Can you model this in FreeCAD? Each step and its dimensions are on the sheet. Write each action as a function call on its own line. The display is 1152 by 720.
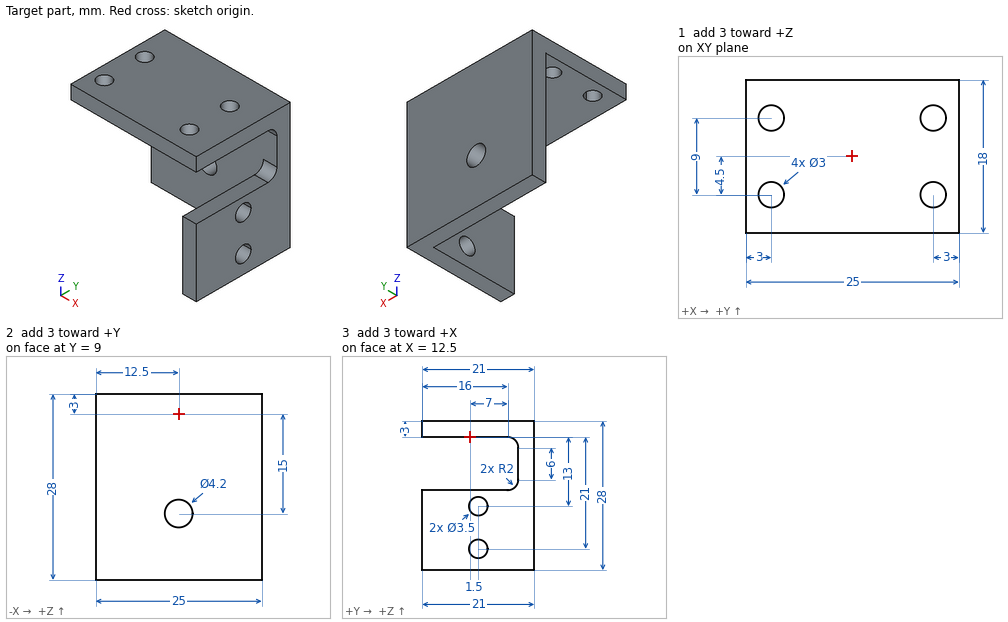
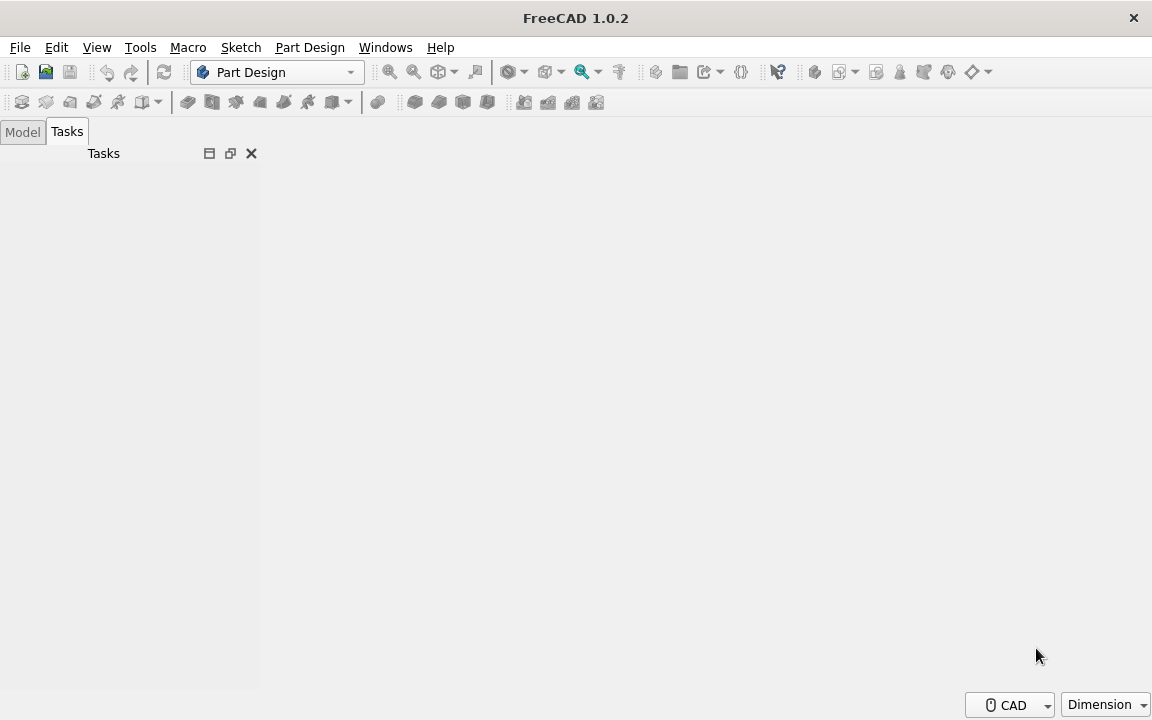
key(ctrl+n)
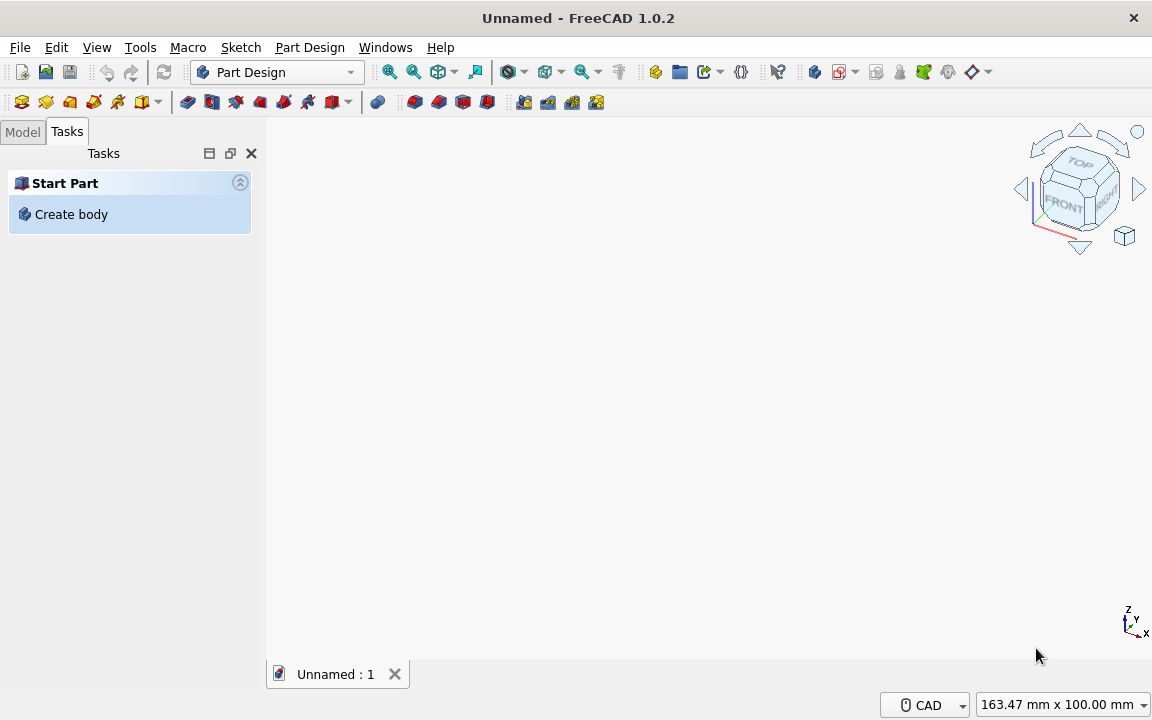
click(840, 72)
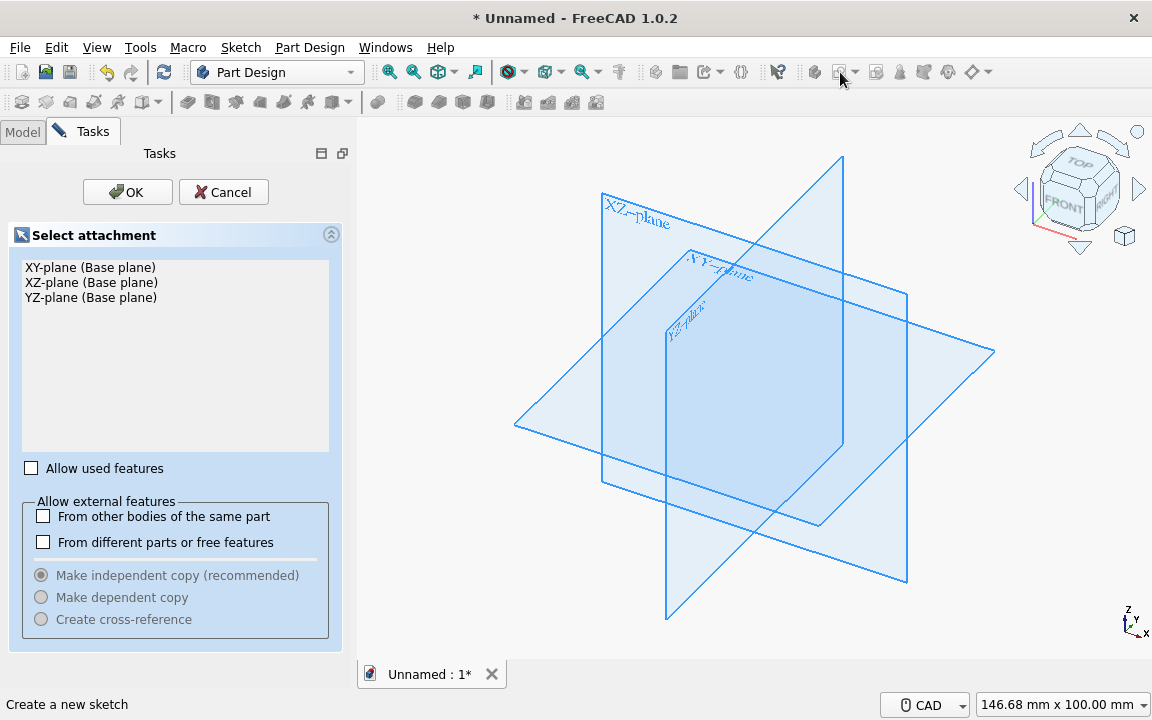
click(82, 268)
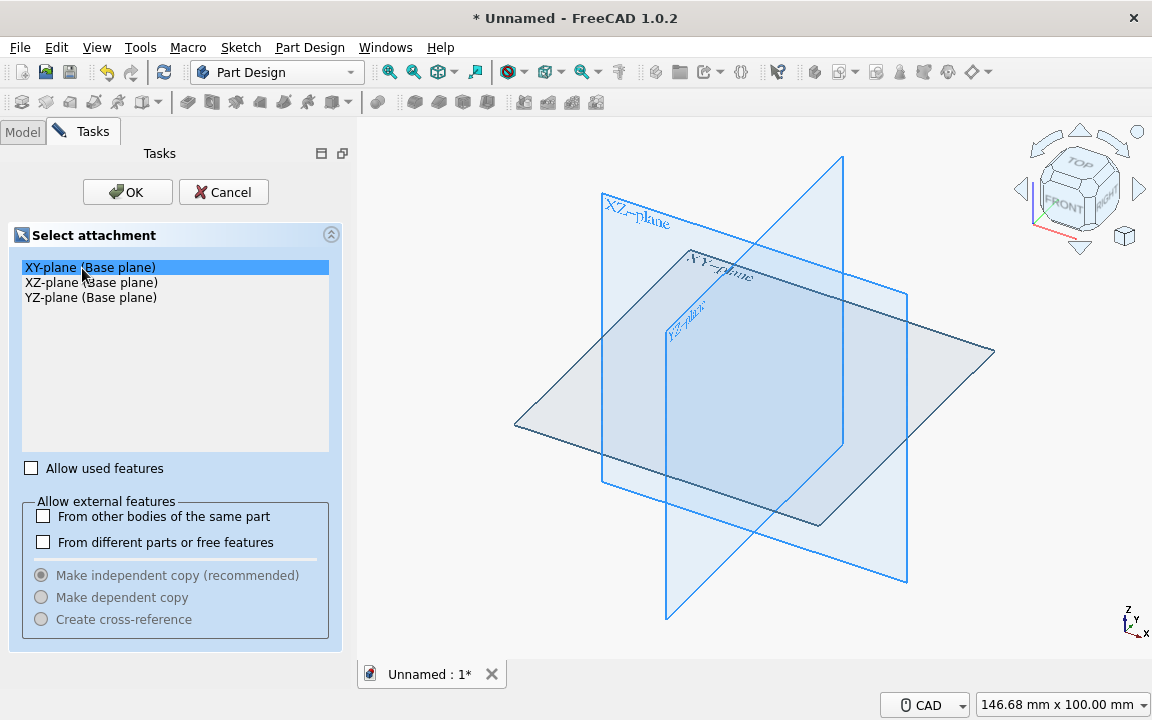
click(128, 192)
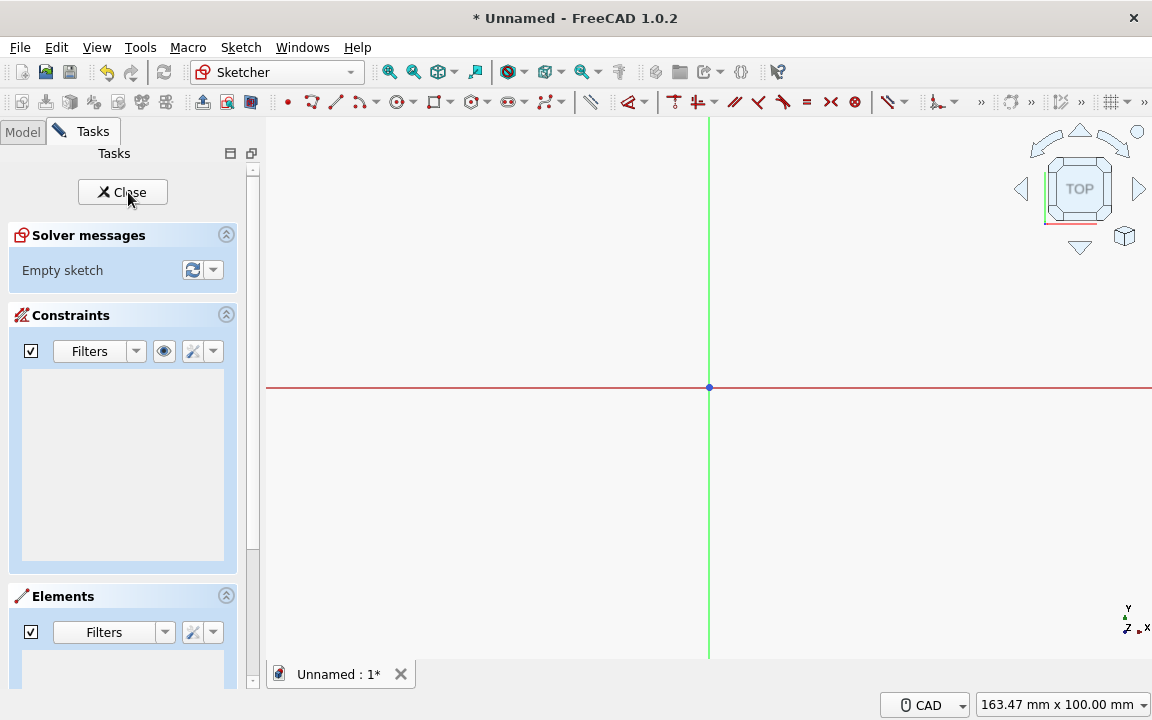
scroll(739, 388, up, 6)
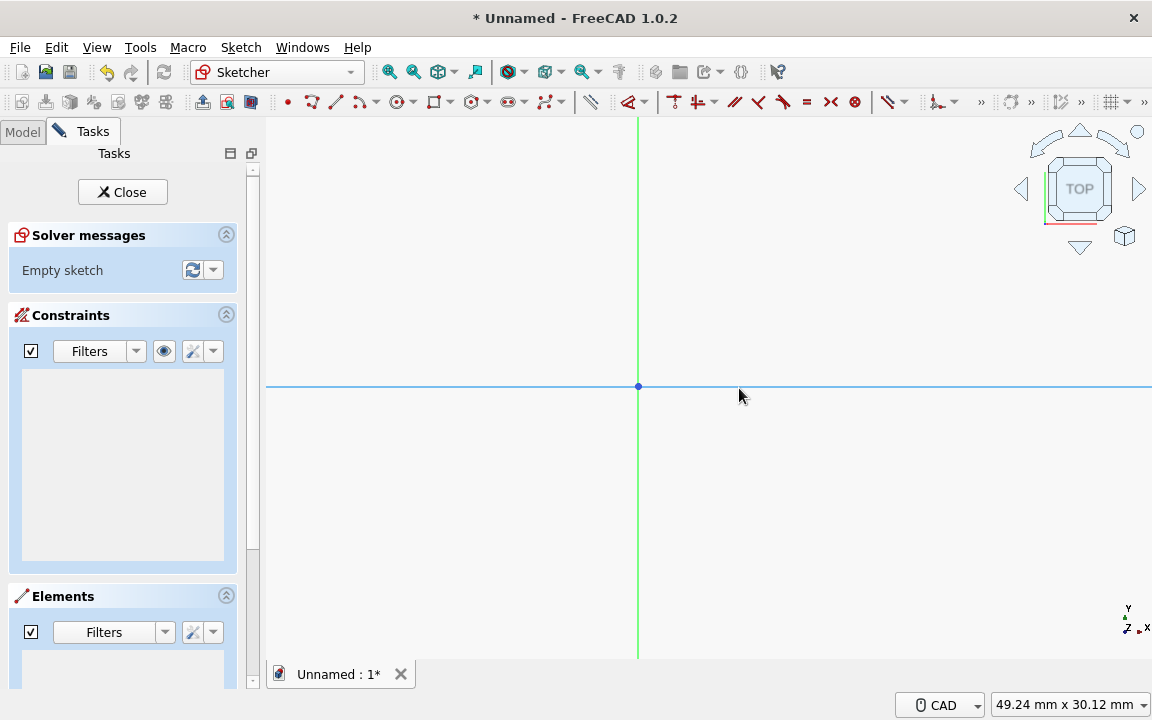
key(g)
key(v)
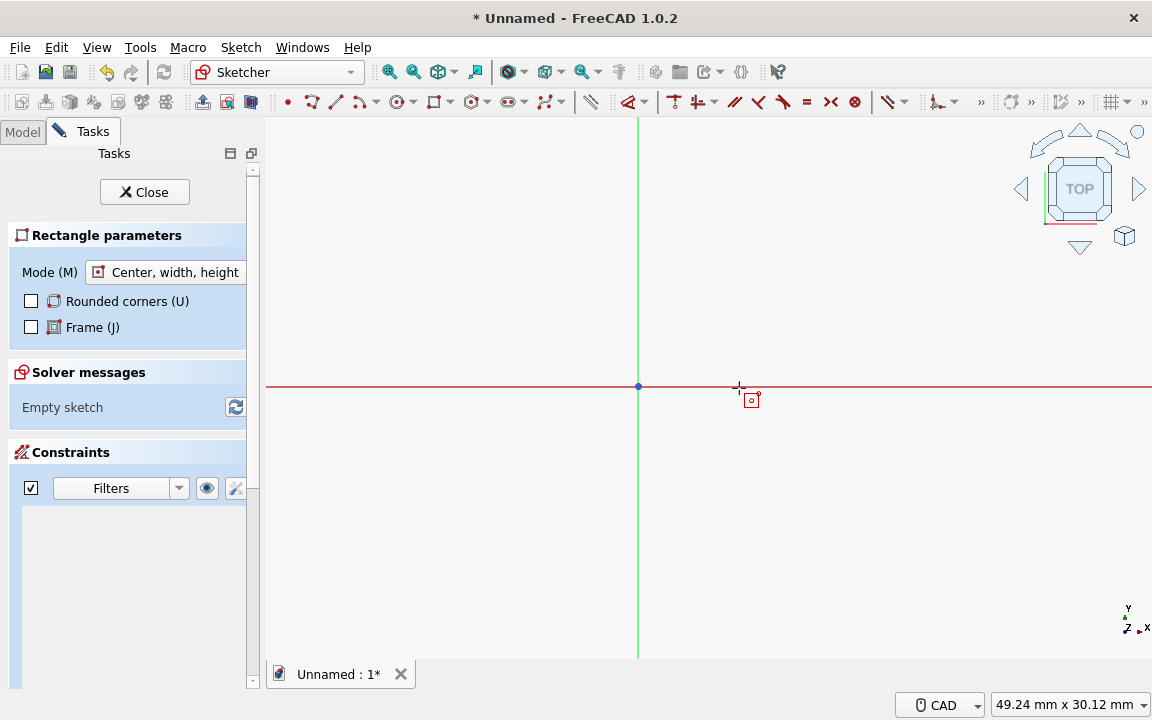
click(638, 387)
click(863, 225)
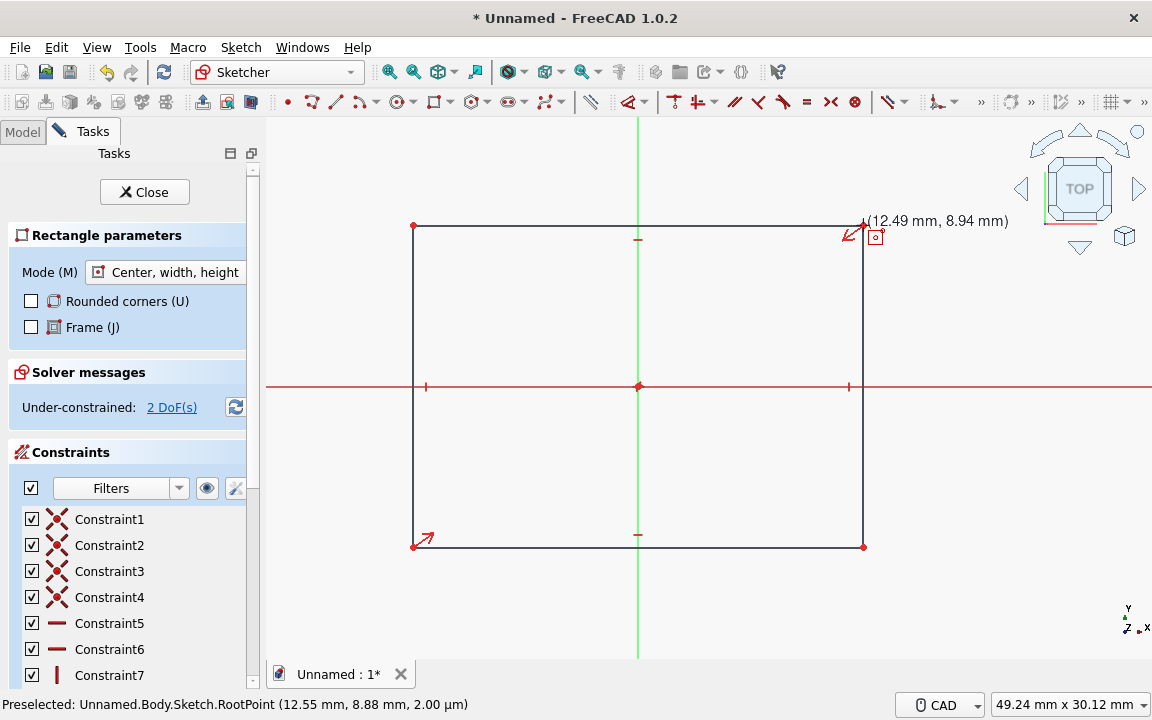
key(g)
key(c)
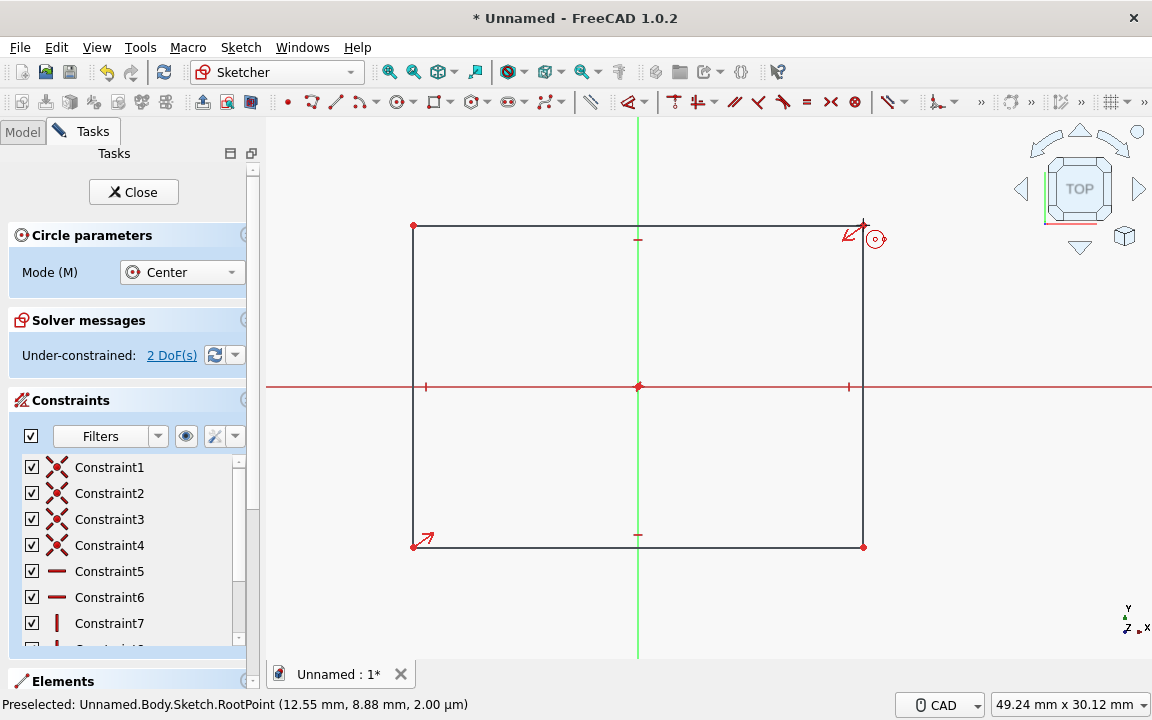
click(467, 468)
click(486, 449)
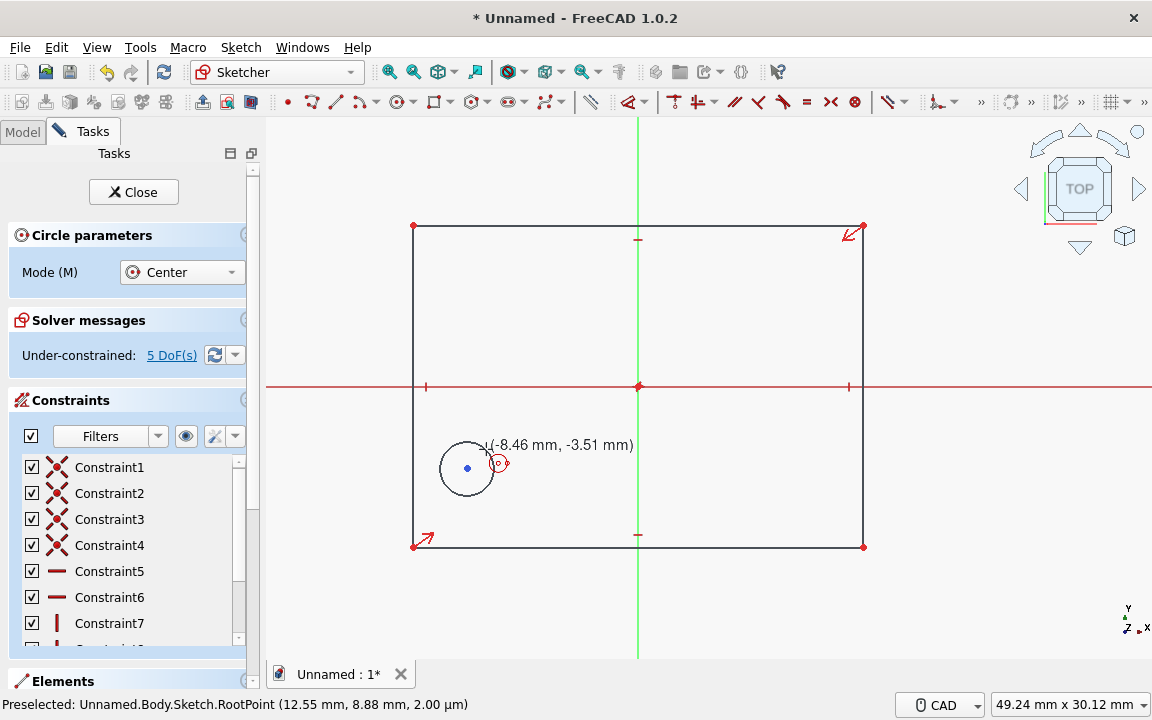
click(809, 468)
click(828, 449)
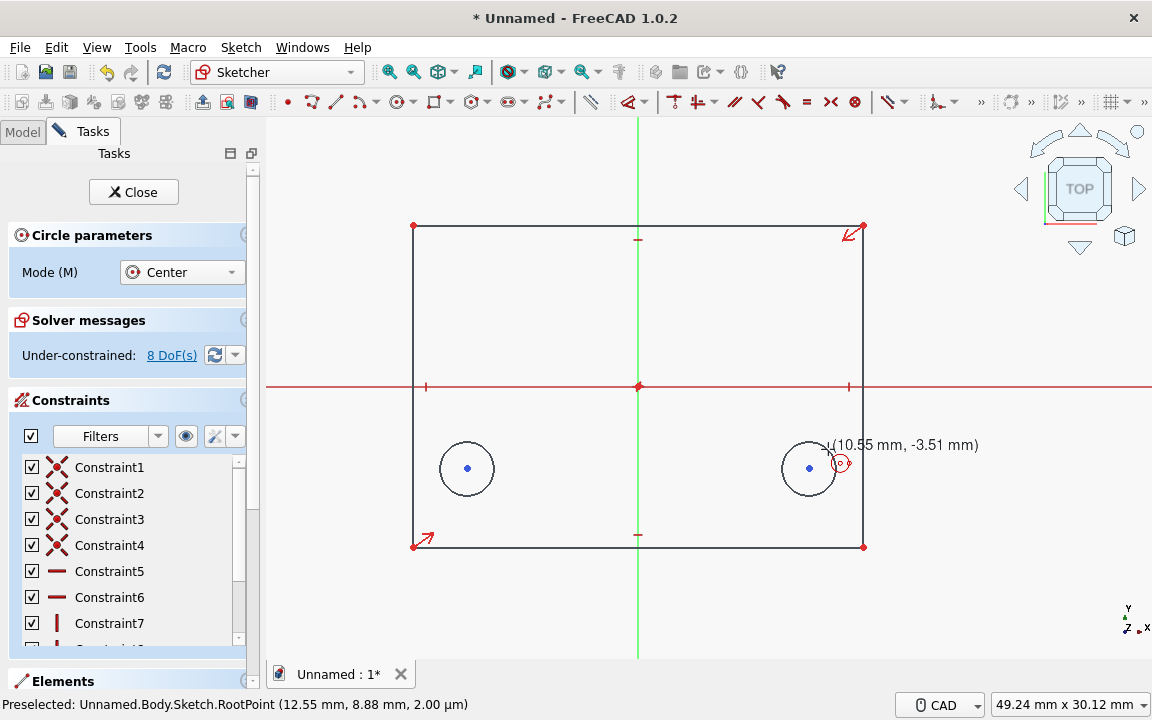
click(467, 306)
click(486, 287)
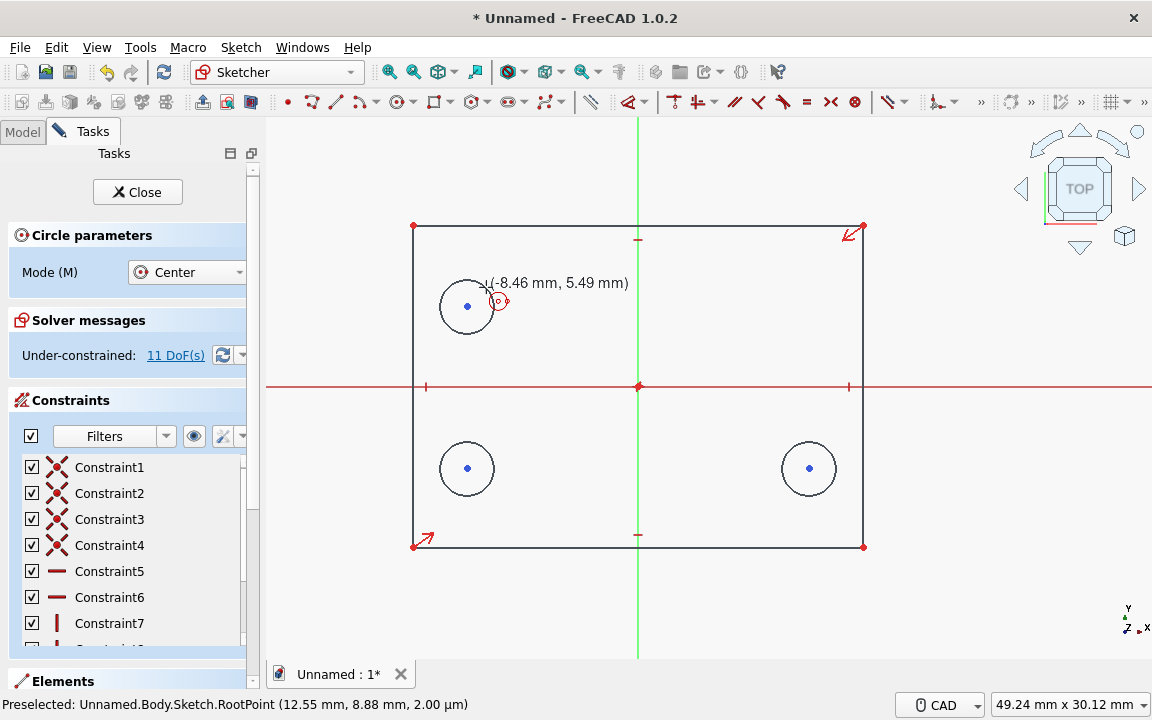
click(809, 306)
click(828, 287)
key(Escape)